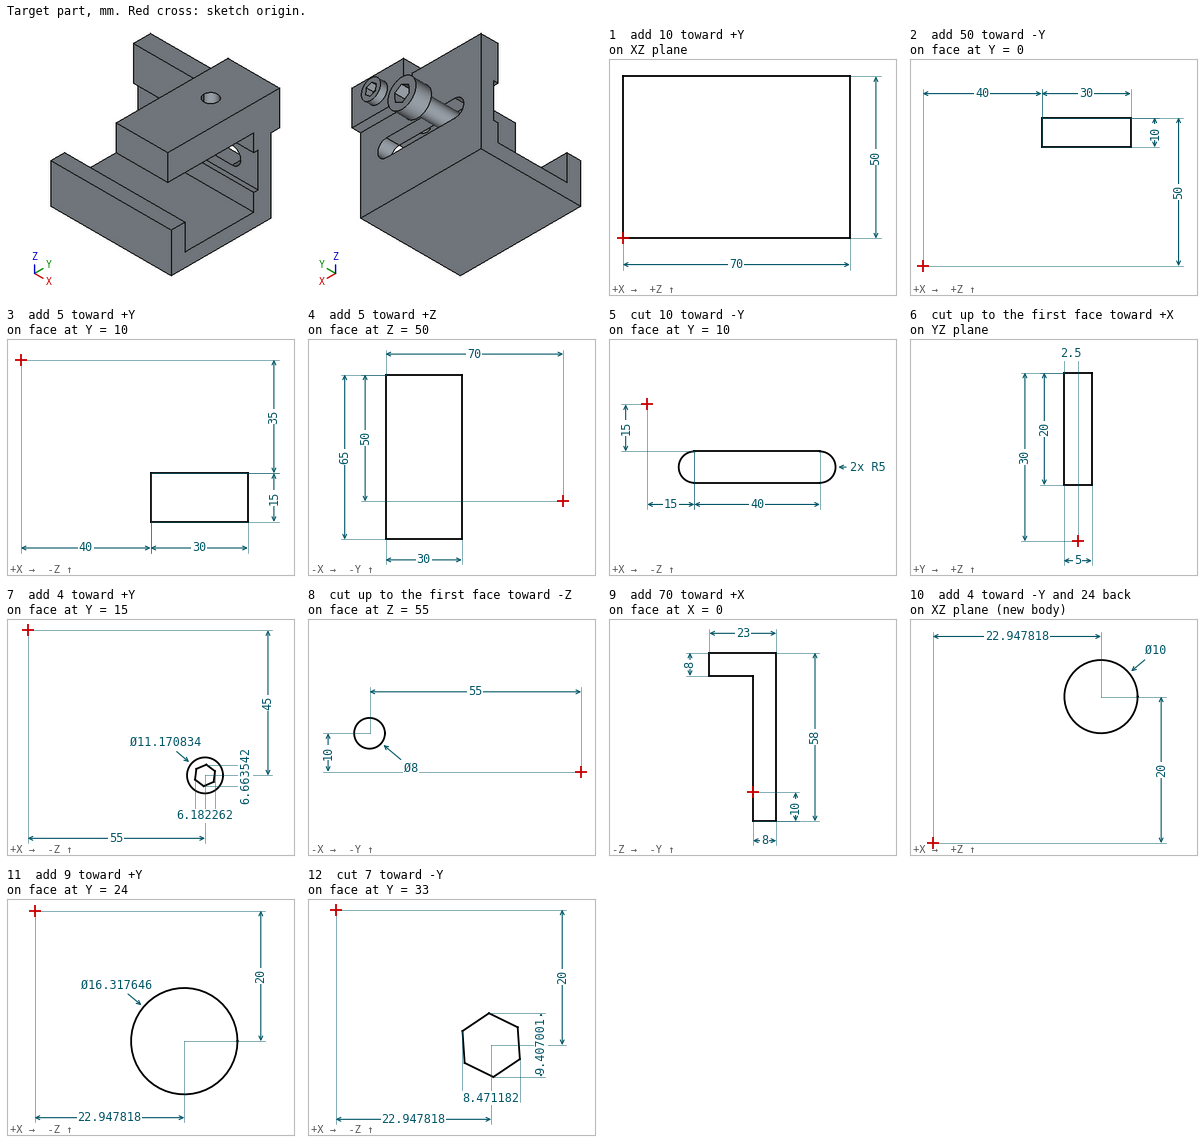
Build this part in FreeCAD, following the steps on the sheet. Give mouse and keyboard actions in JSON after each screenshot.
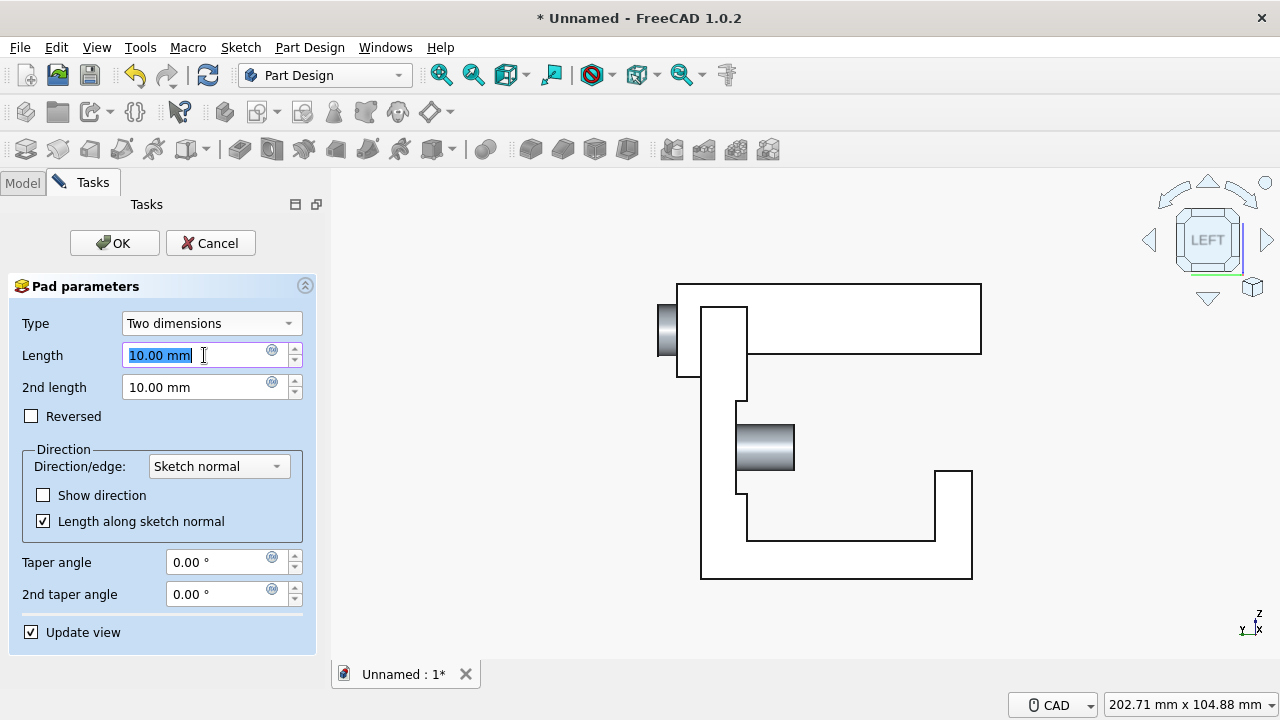
{"action": "type", "text": "4"}
{"action": "key", "text": "Tab"}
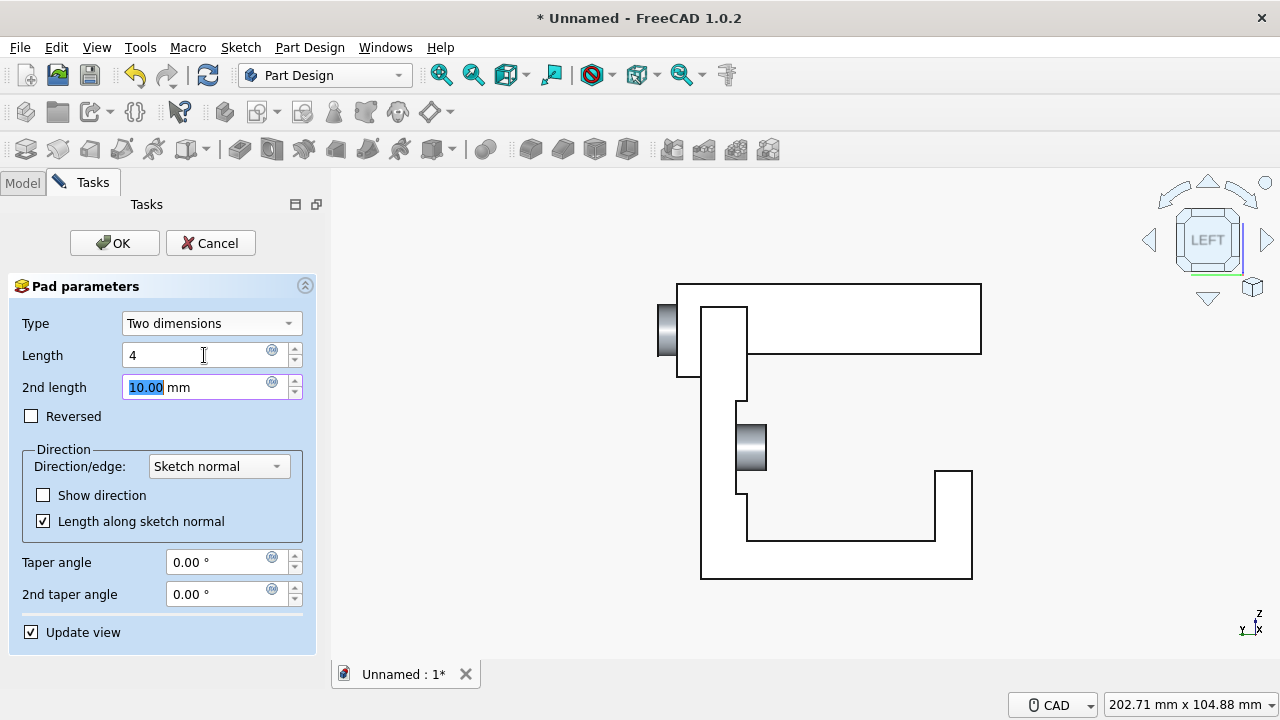
{"action": "type", "text": "24"}
{"action": "key", "text": "Tab"}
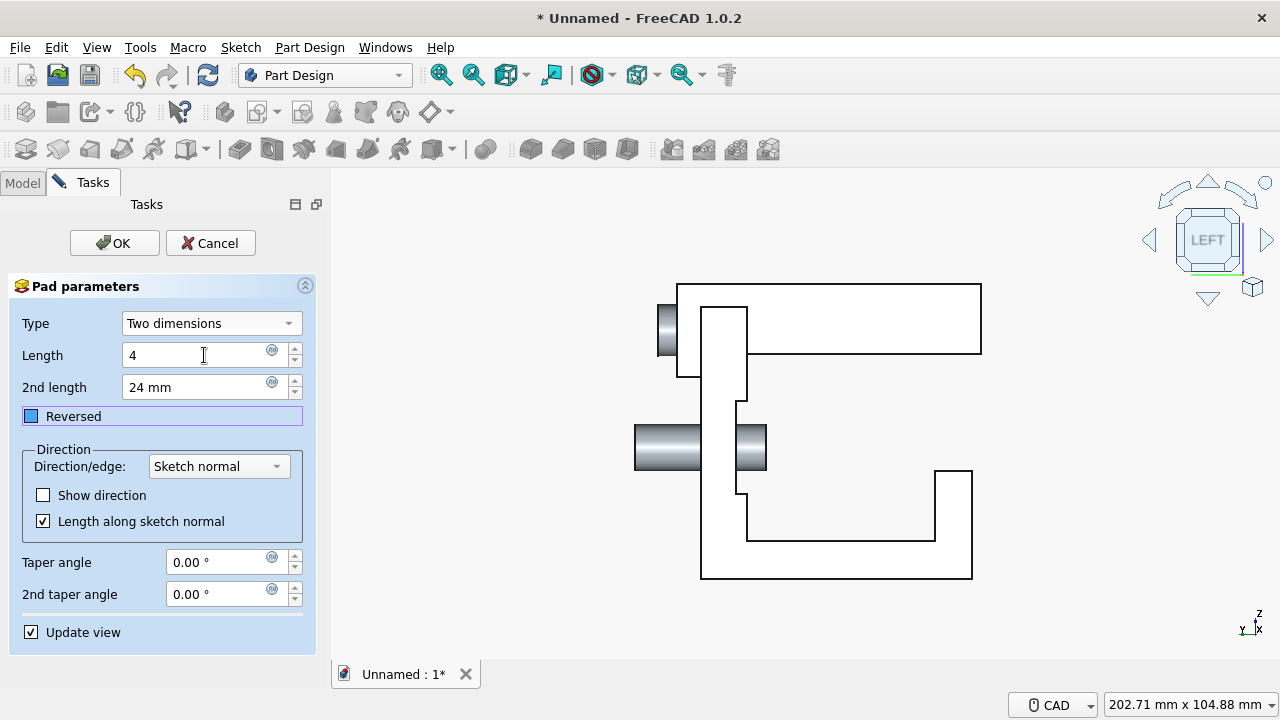
{"action": "left_click", "coordinate": [115, 243]}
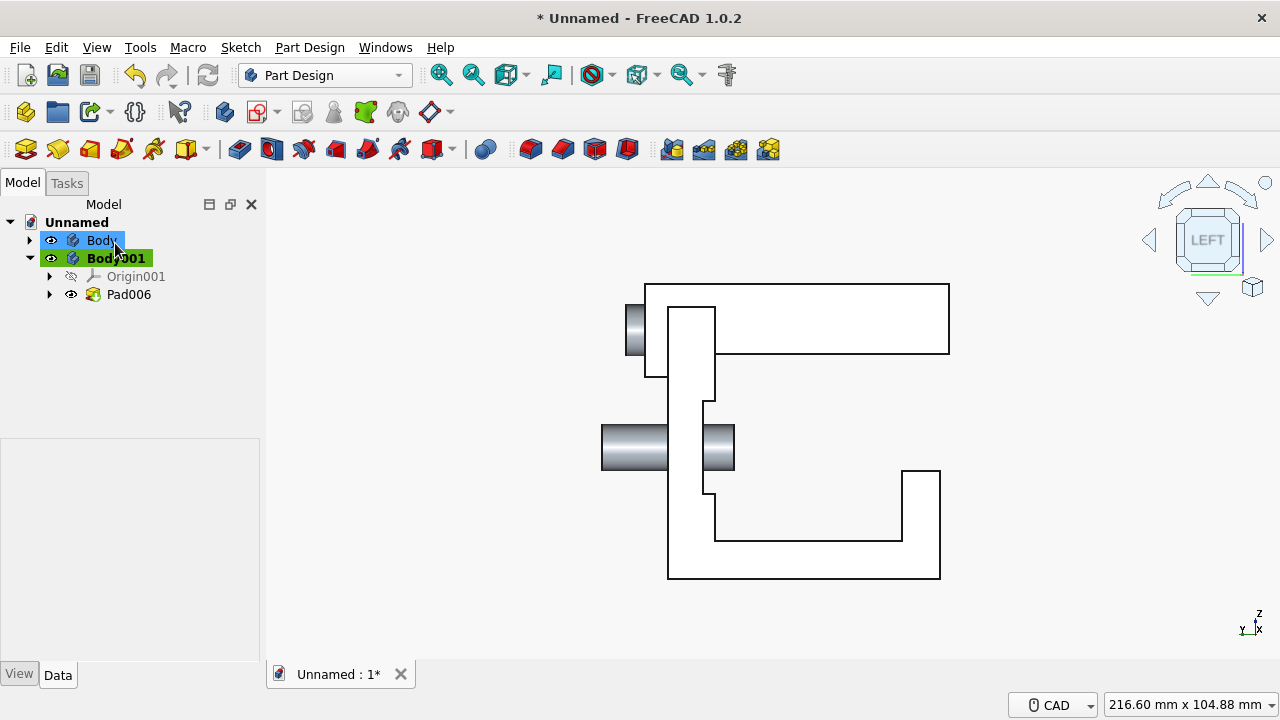
{"action": "left_click", "coordinate": [442, 76]}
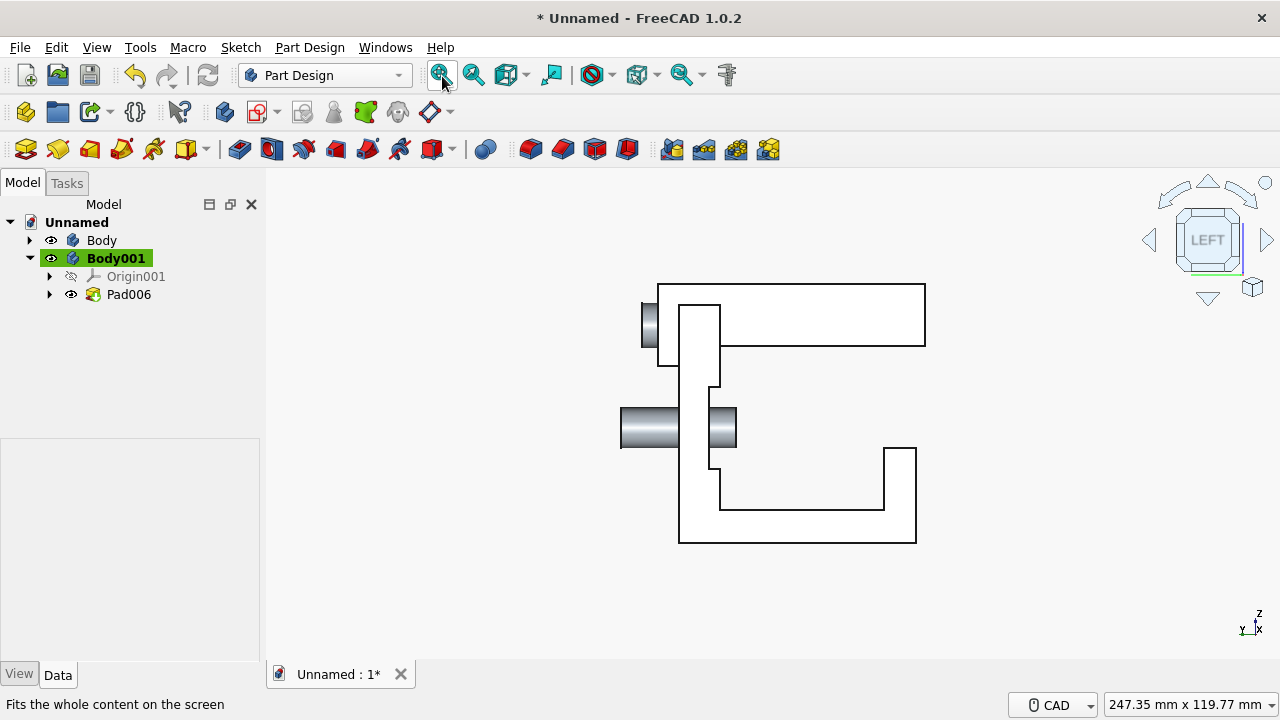
{"action": "key", "text": "4"}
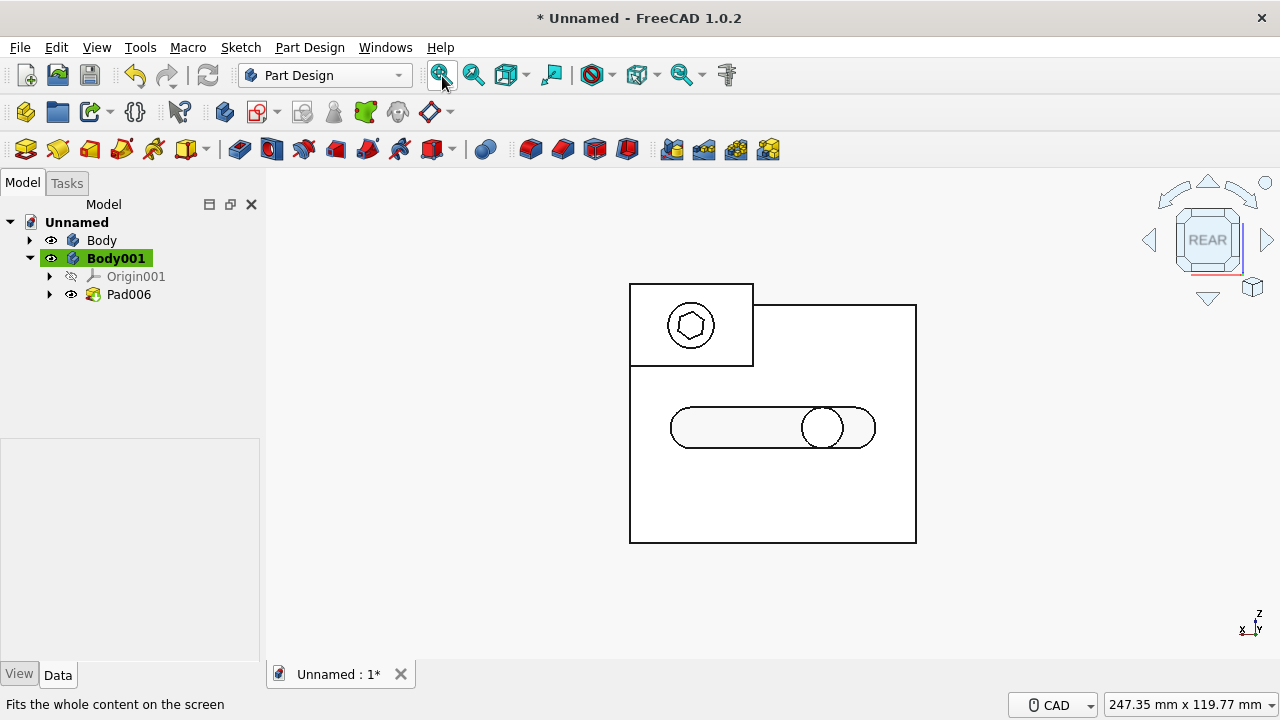
{"action": "left_click", "coordinate": [442, 76]}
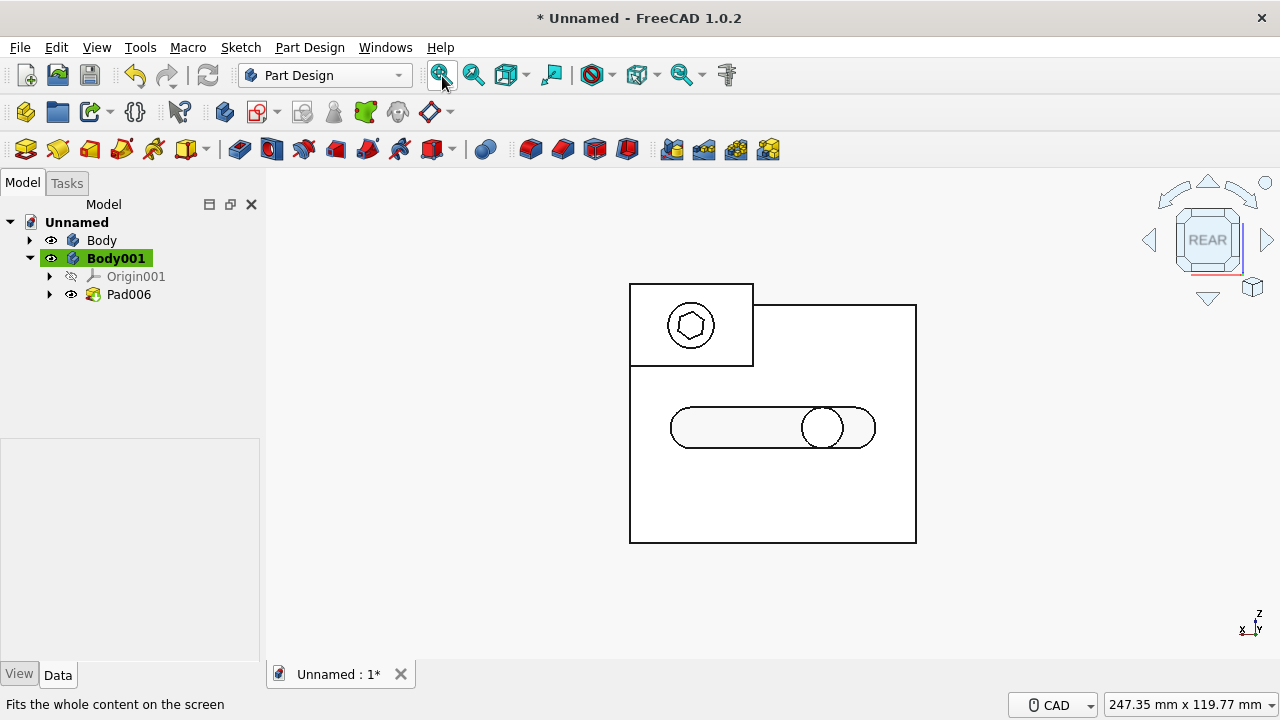
{"action": "left_click", "coordinate": [822, 427]}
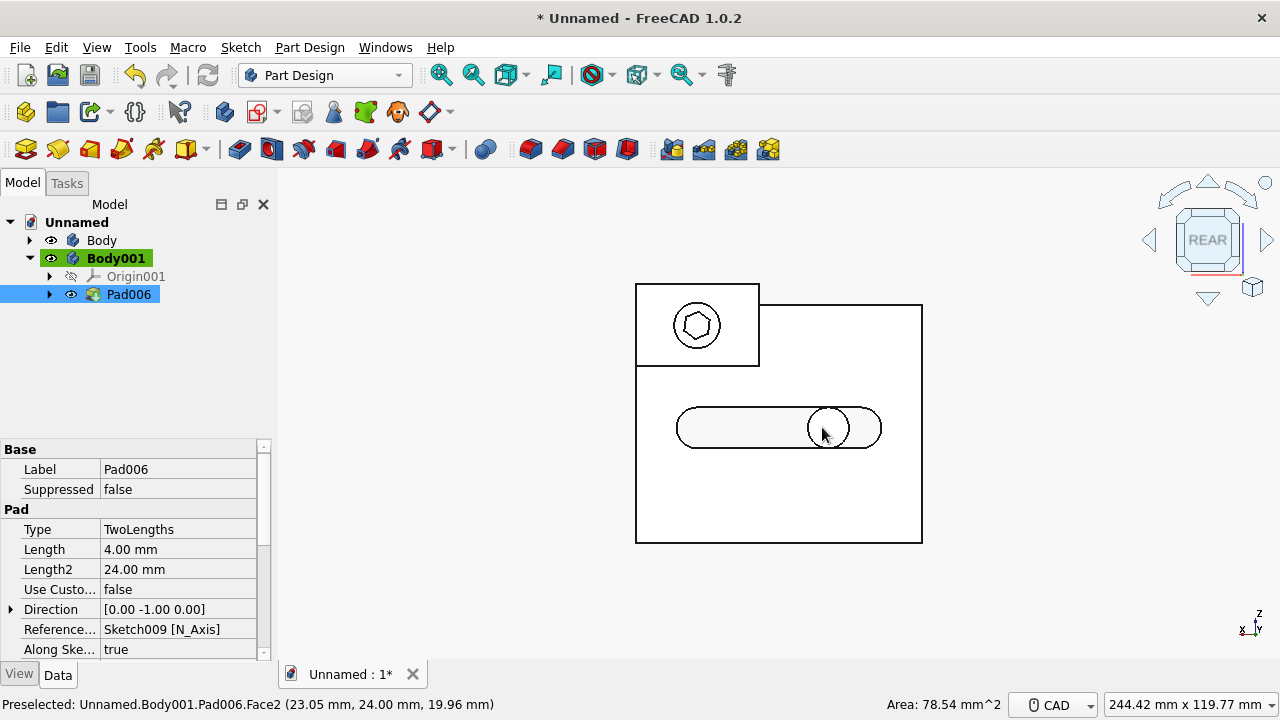
{"action": "left_click", "coordinate": [258, 112]}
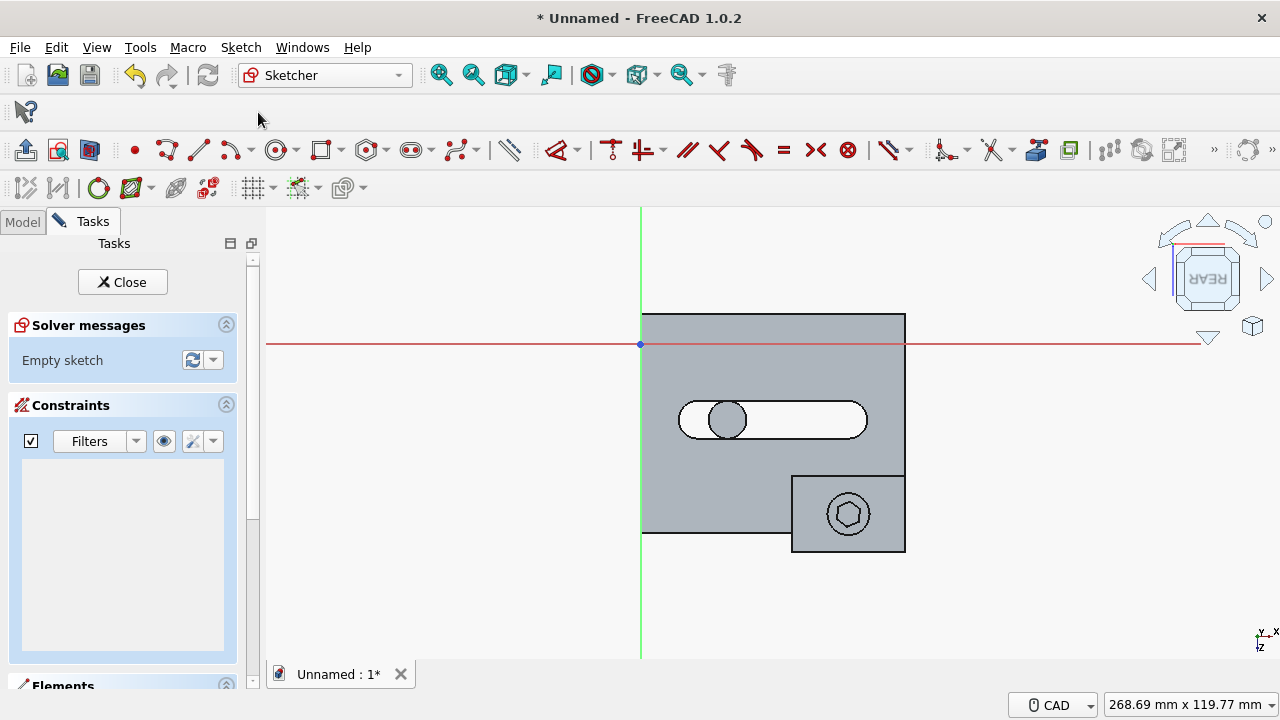
{"action": "scroll", "coordinate": [697, 377], "scroll_direction": "up", "scroll_amount": 5}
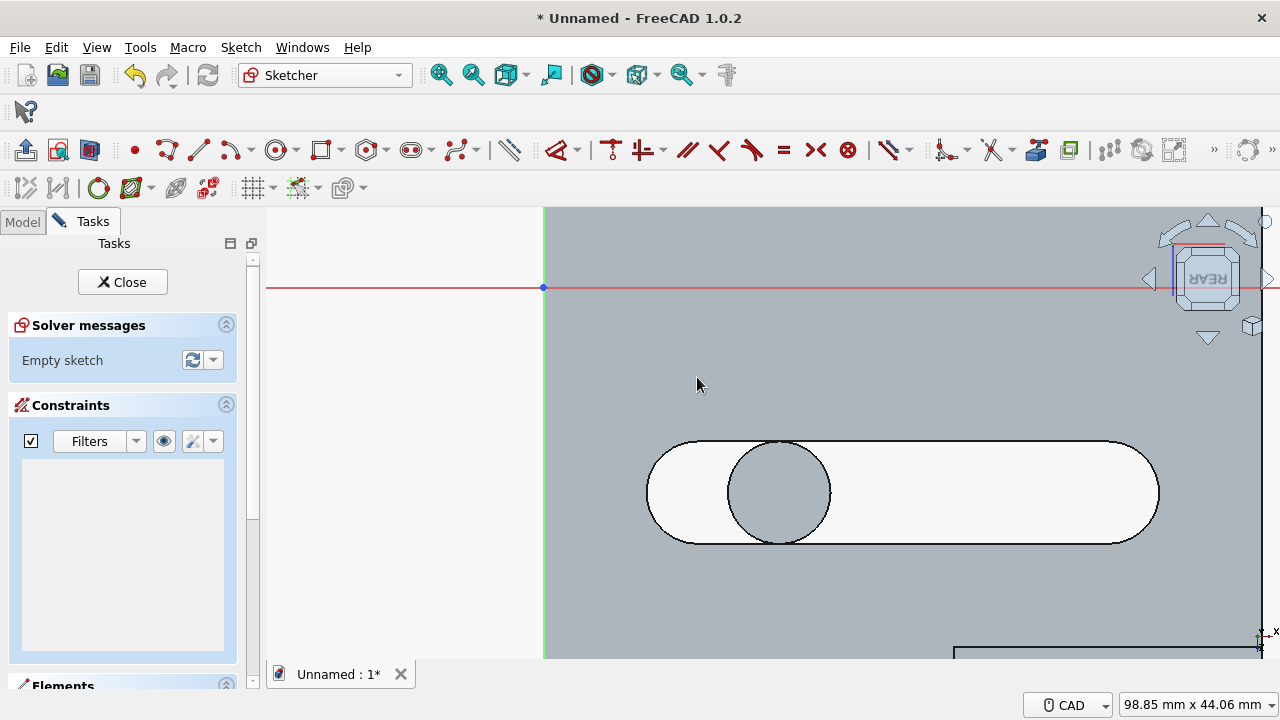
{"action": "left_click", "coordinate": [276, 150]}